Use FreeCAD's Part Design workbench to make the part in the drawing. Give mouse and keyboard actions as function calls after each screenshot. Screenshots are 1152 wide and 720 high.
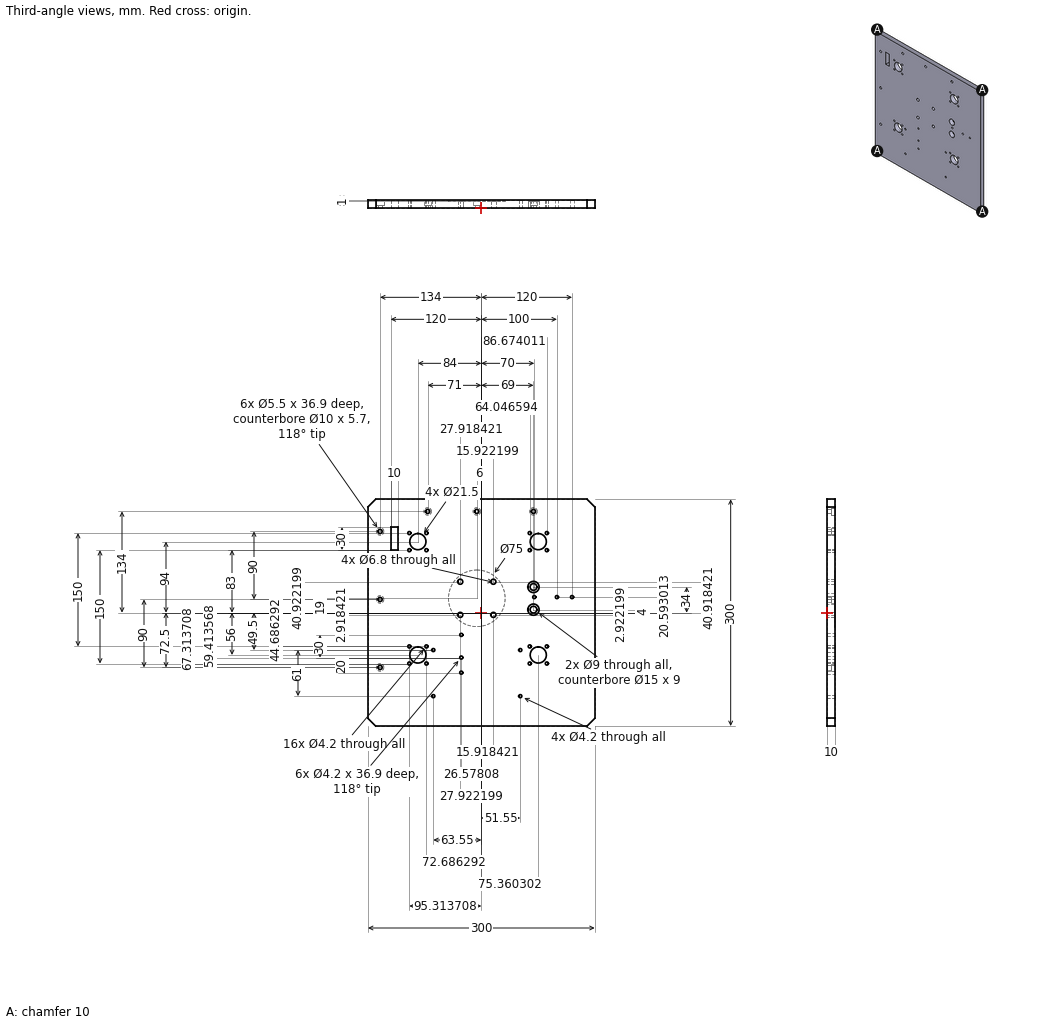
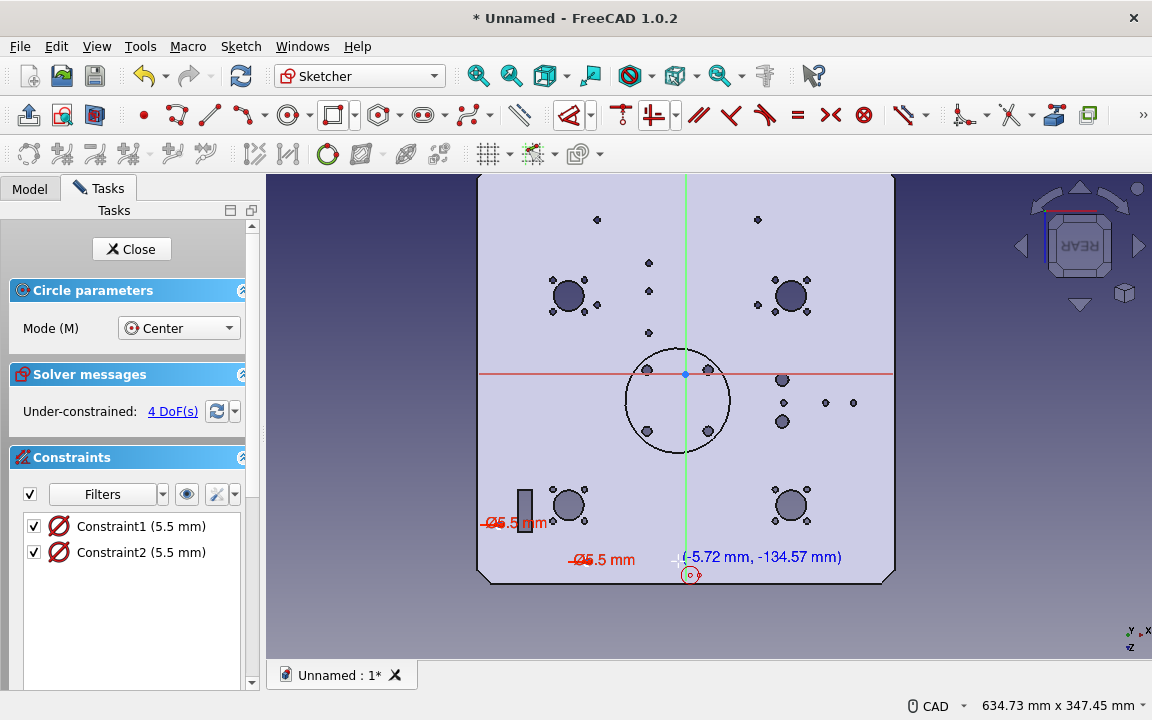
scroll(678, 561, up, 4)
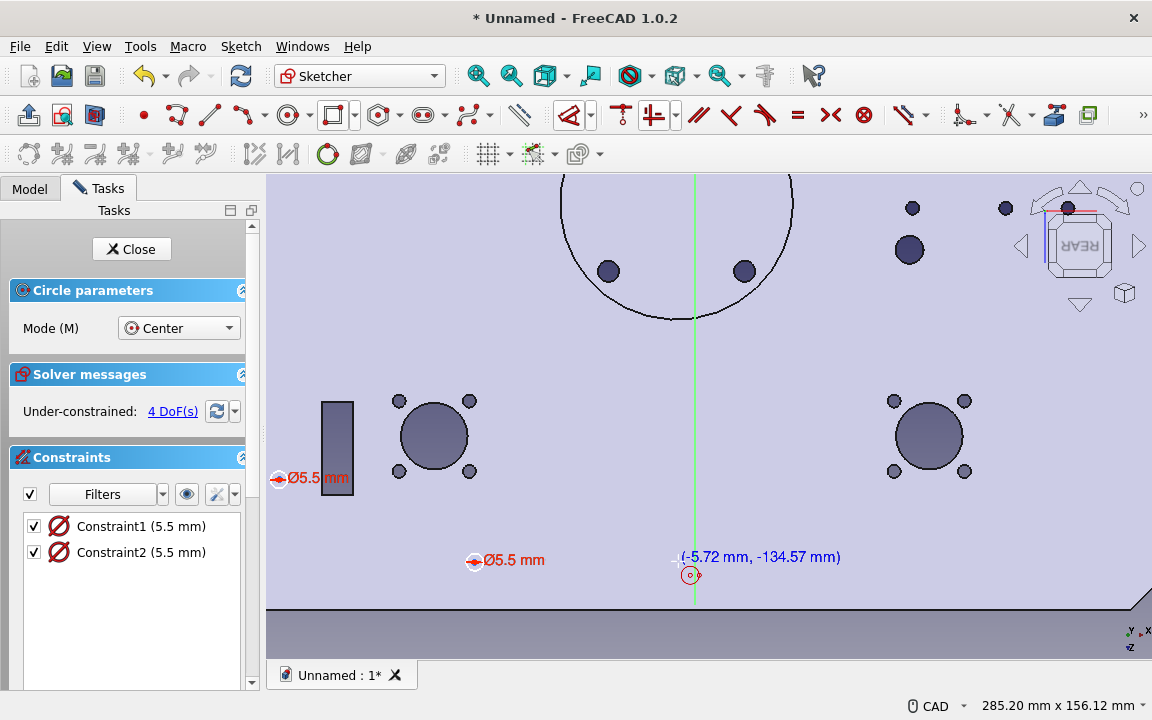
click(677, 560)
move(671, 554)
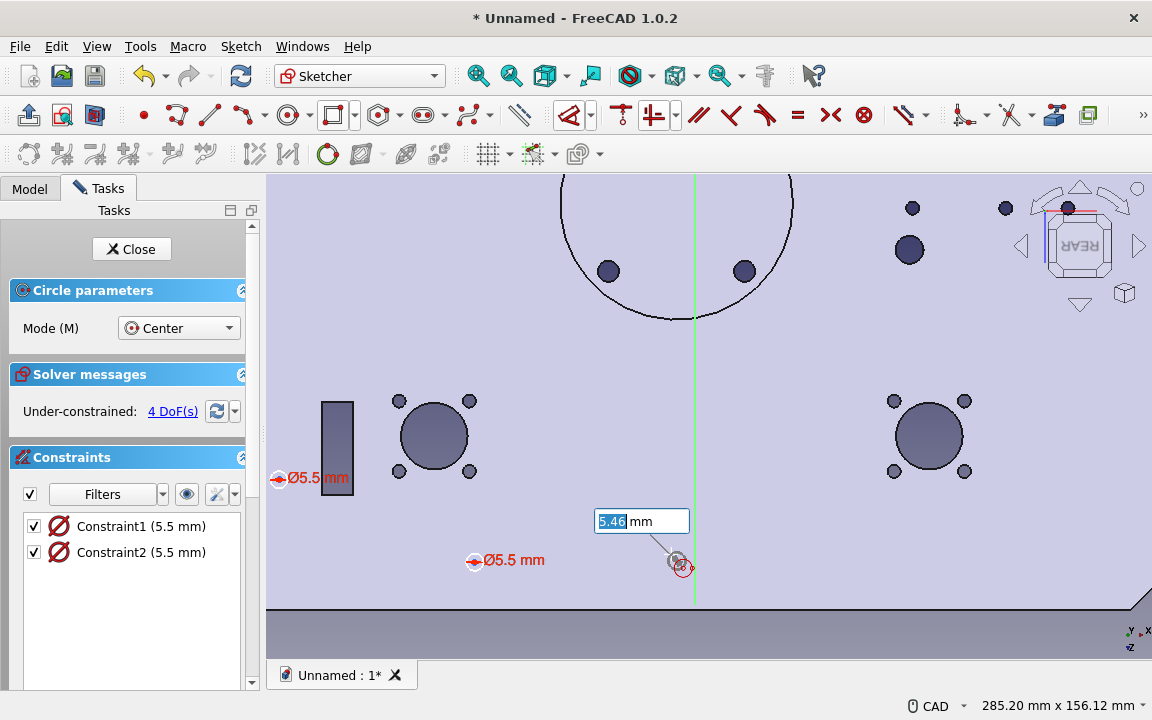
text(5.5)
key(Return)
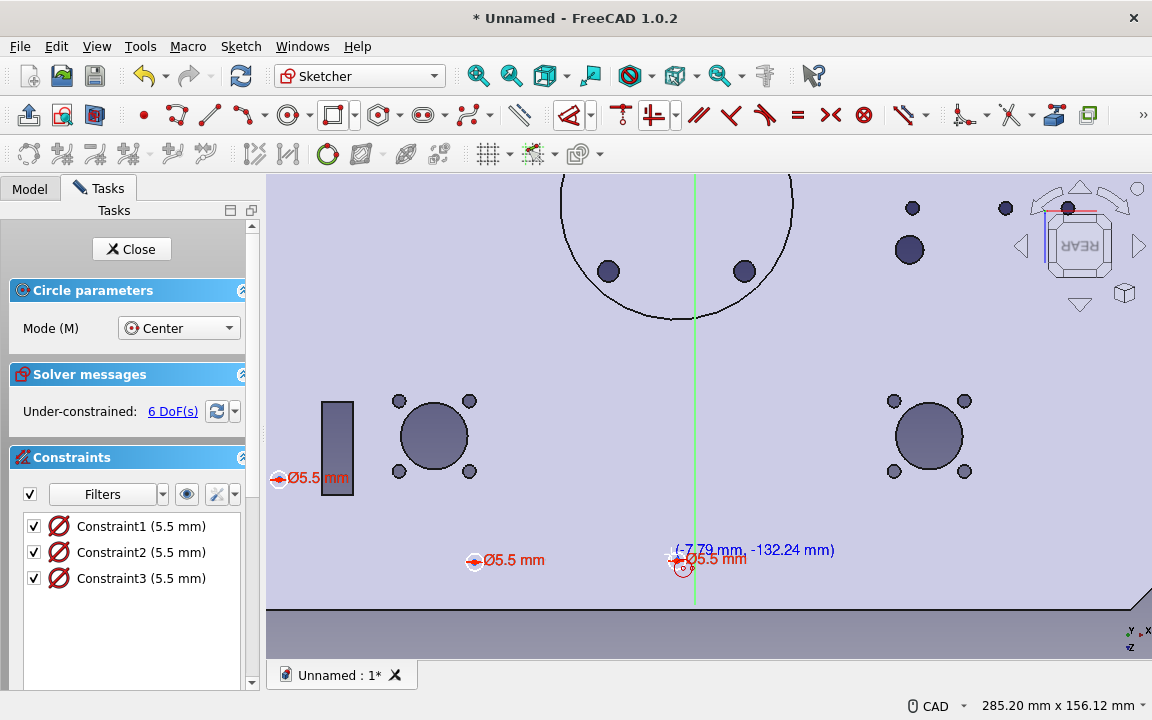
scroll(910, 560, up, 5)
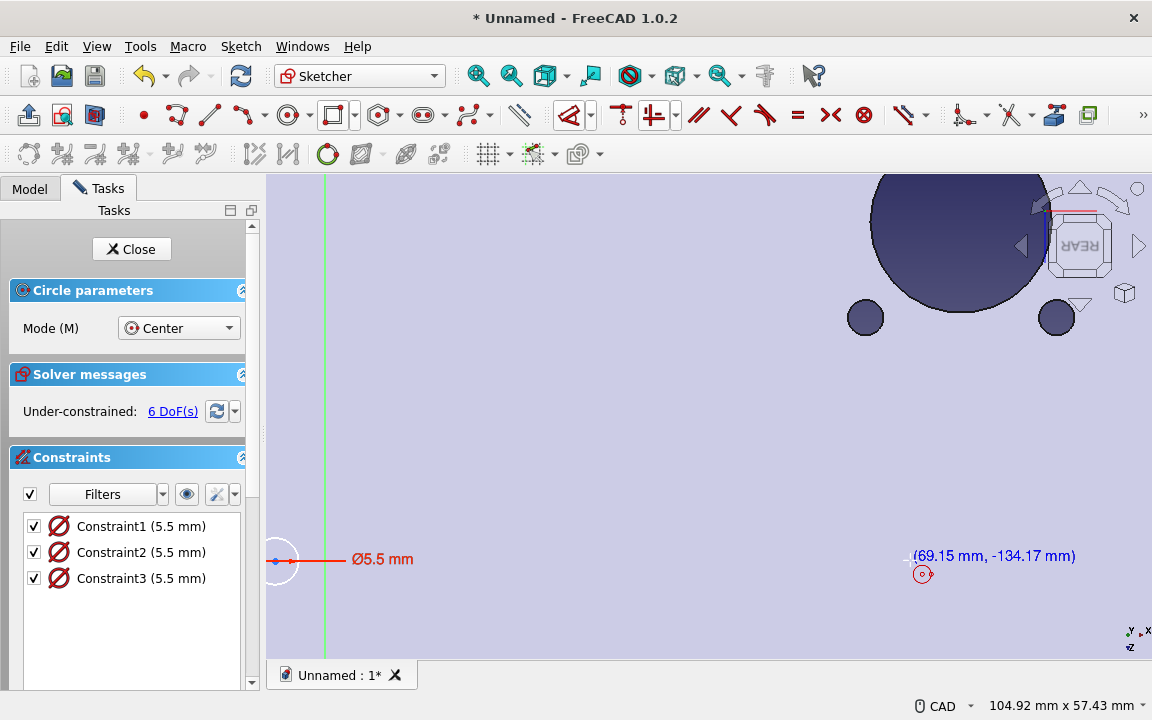
scroll(757, 561, down, 9)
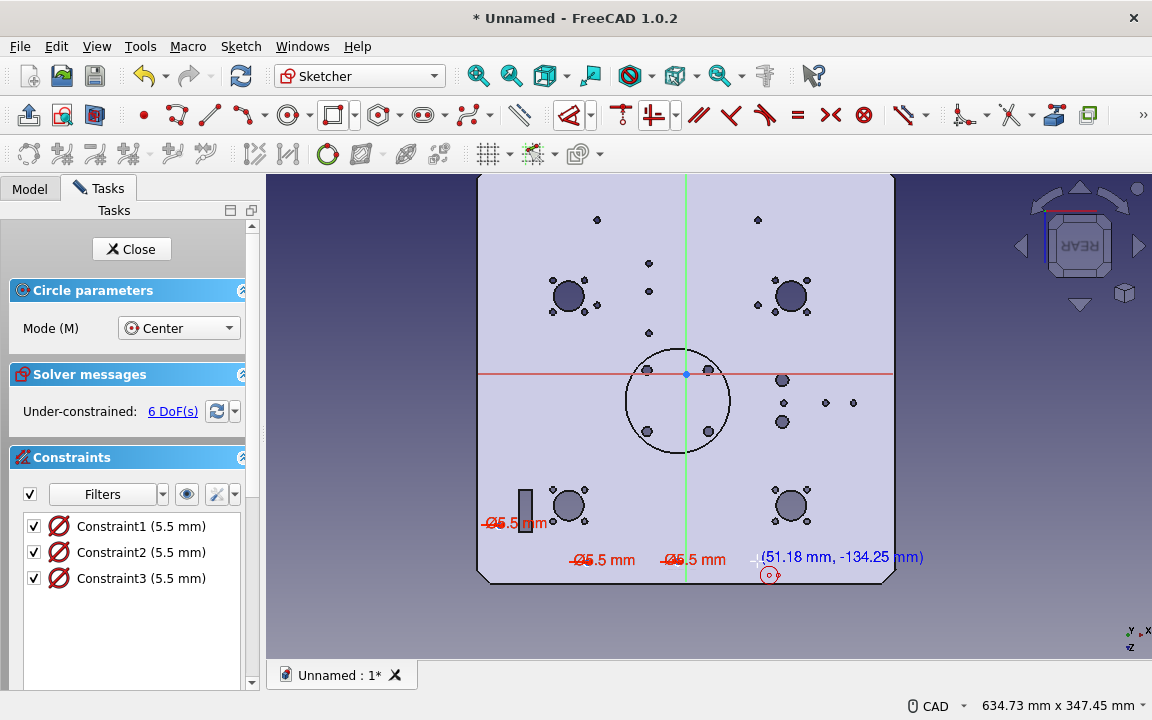
click(782, 561)
move(785, 559)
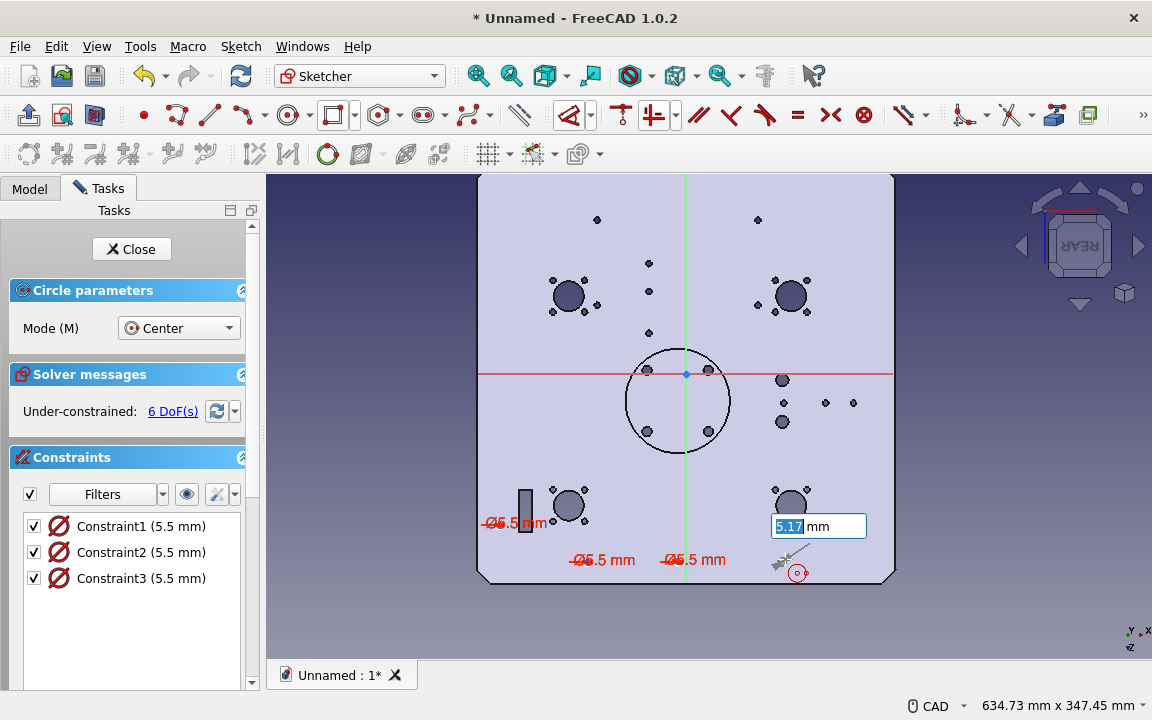
text(5.5)
key(Return)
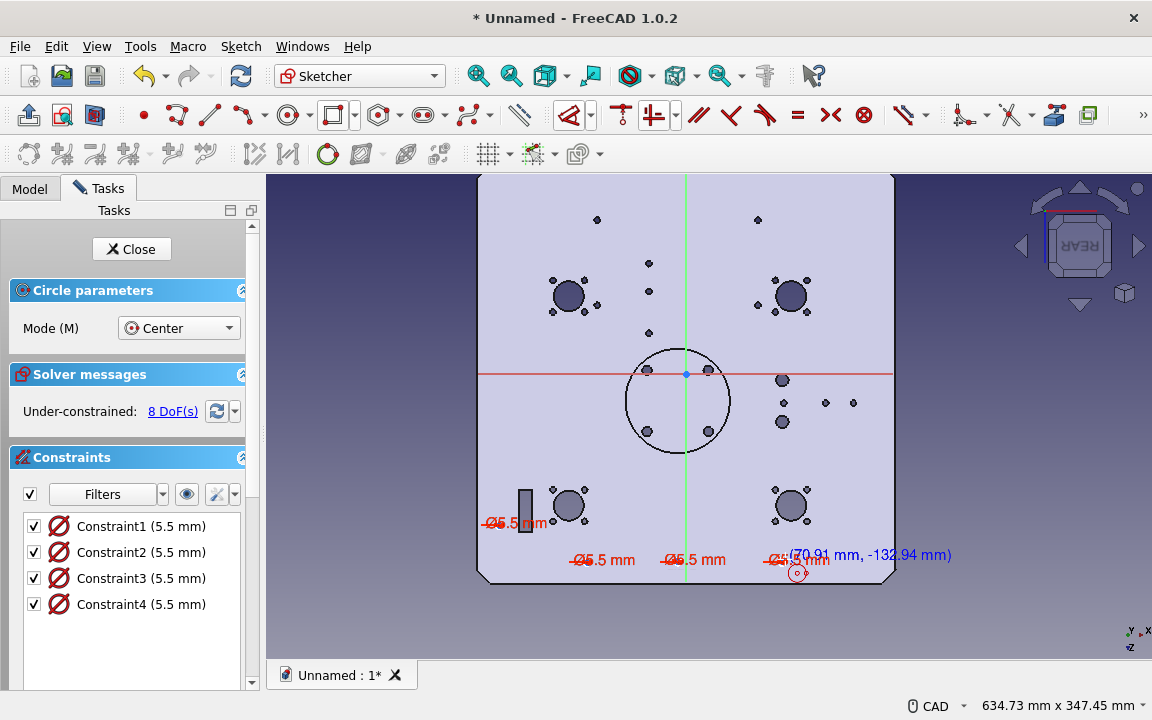
scroll(499, 273, up, 9)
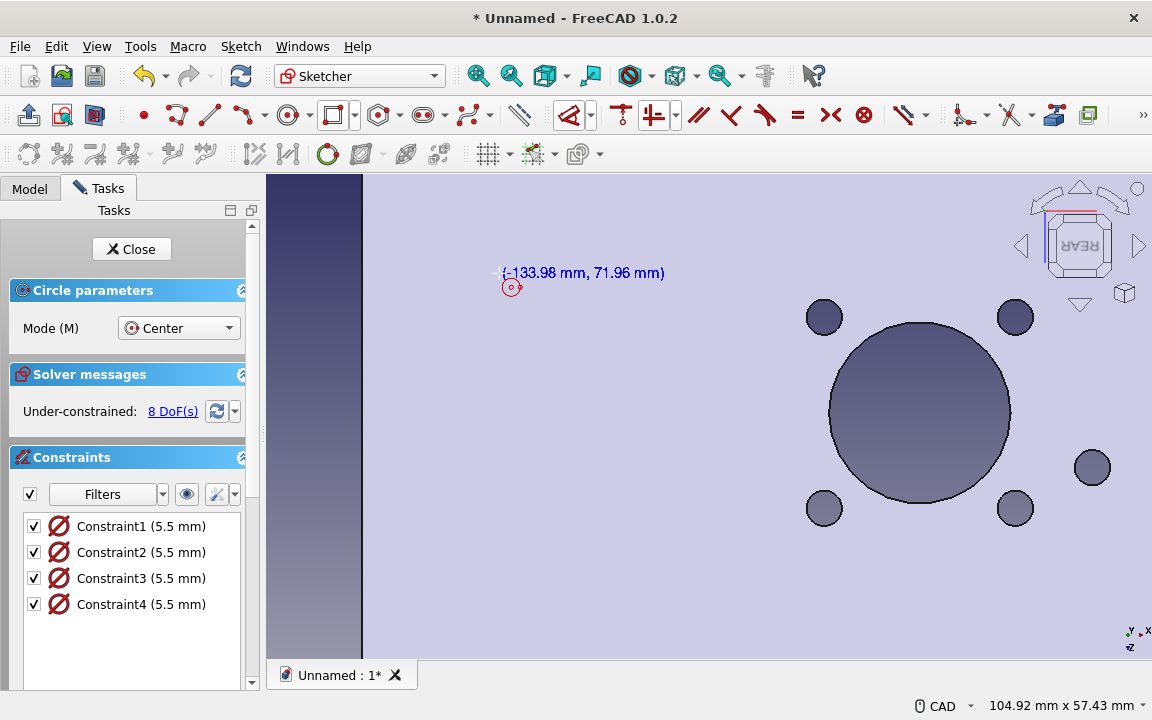
scroll(499, 272, down, 9)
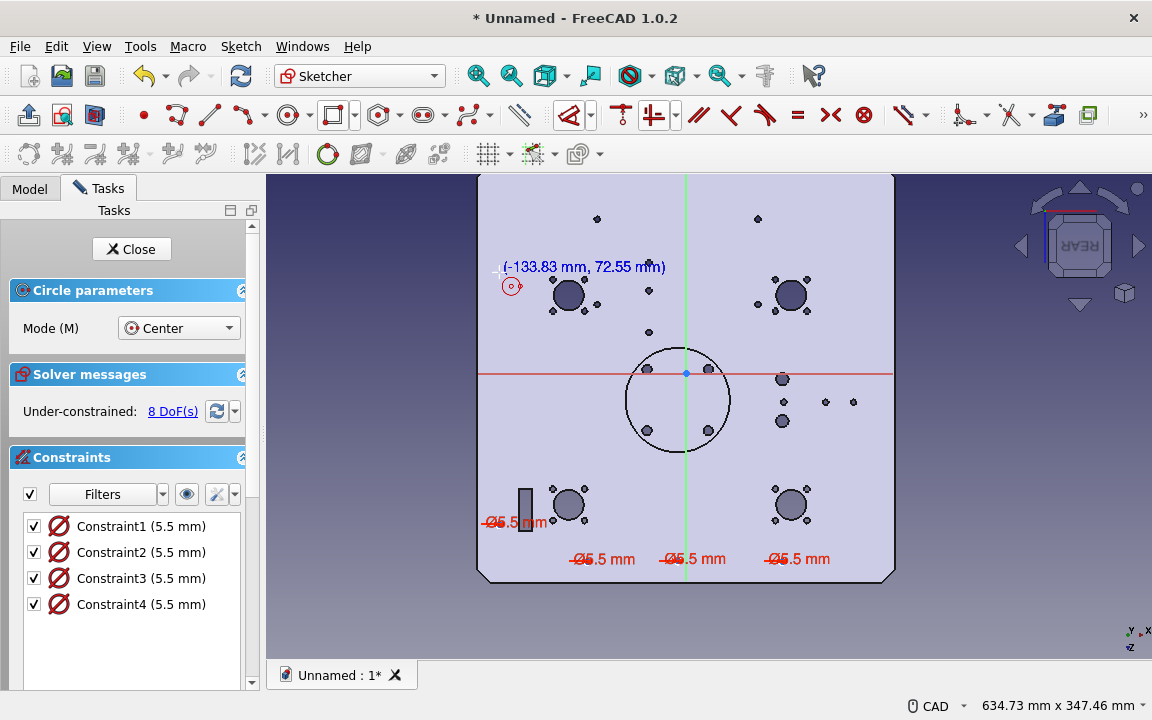
click(499, 272)
move(502, 270)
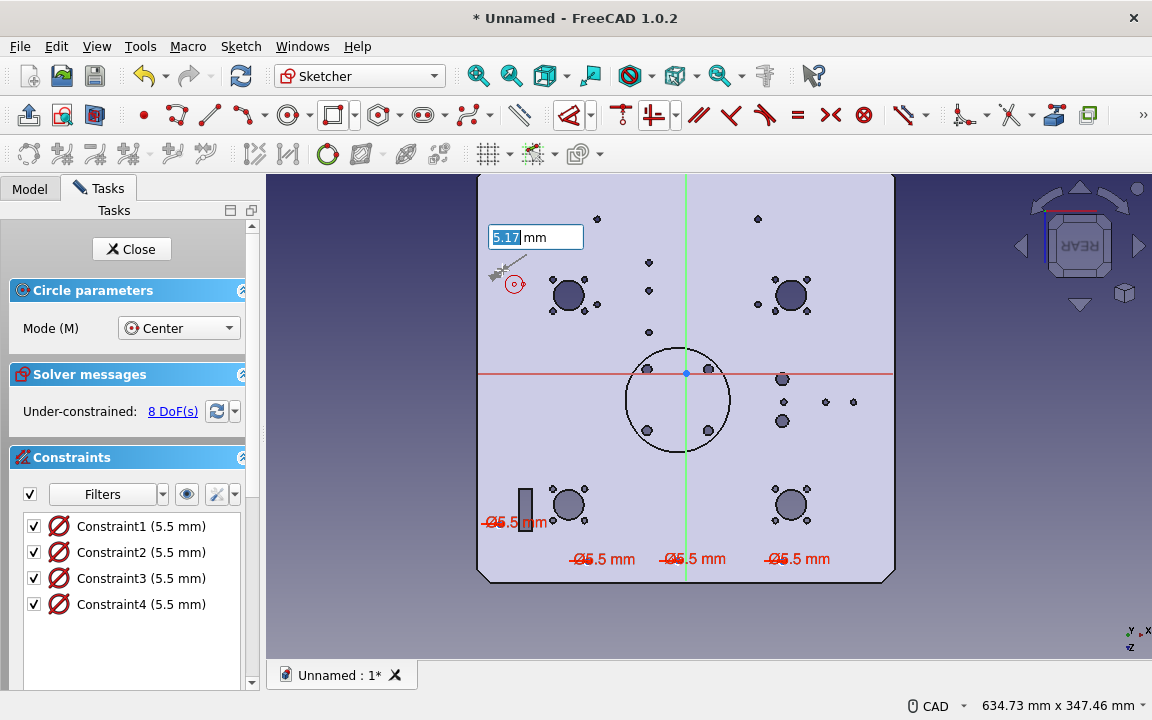
text(5.5)
key(Return)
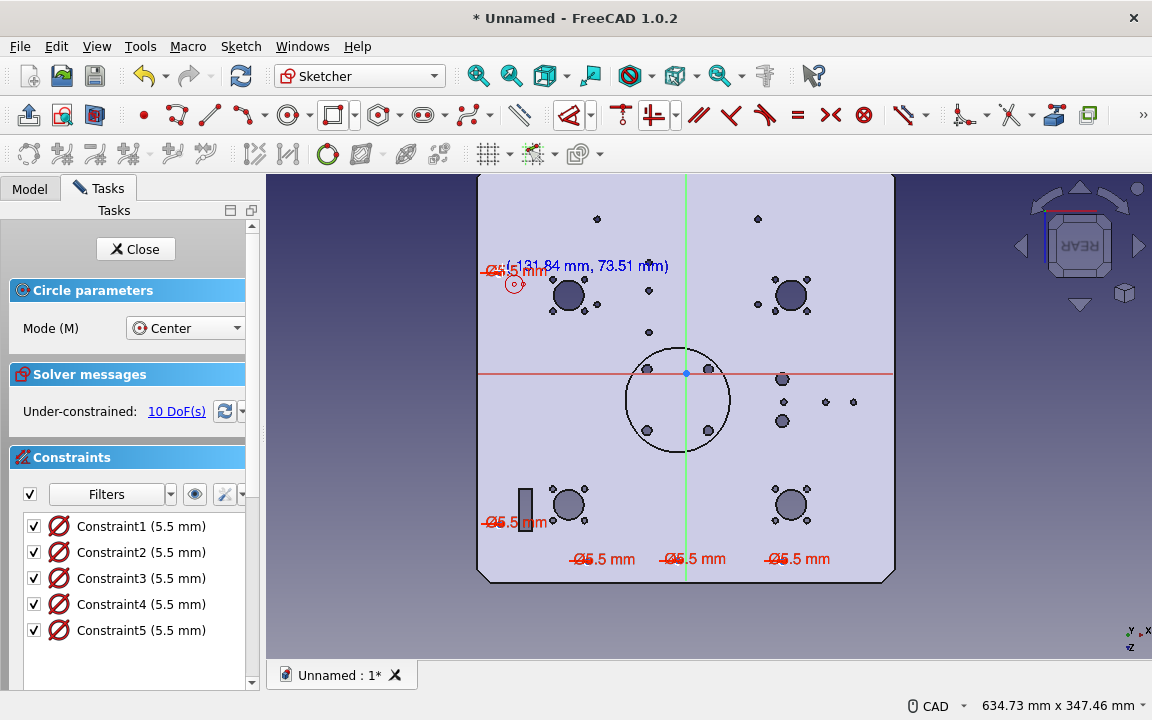
scroll(499, 398, up, 9)